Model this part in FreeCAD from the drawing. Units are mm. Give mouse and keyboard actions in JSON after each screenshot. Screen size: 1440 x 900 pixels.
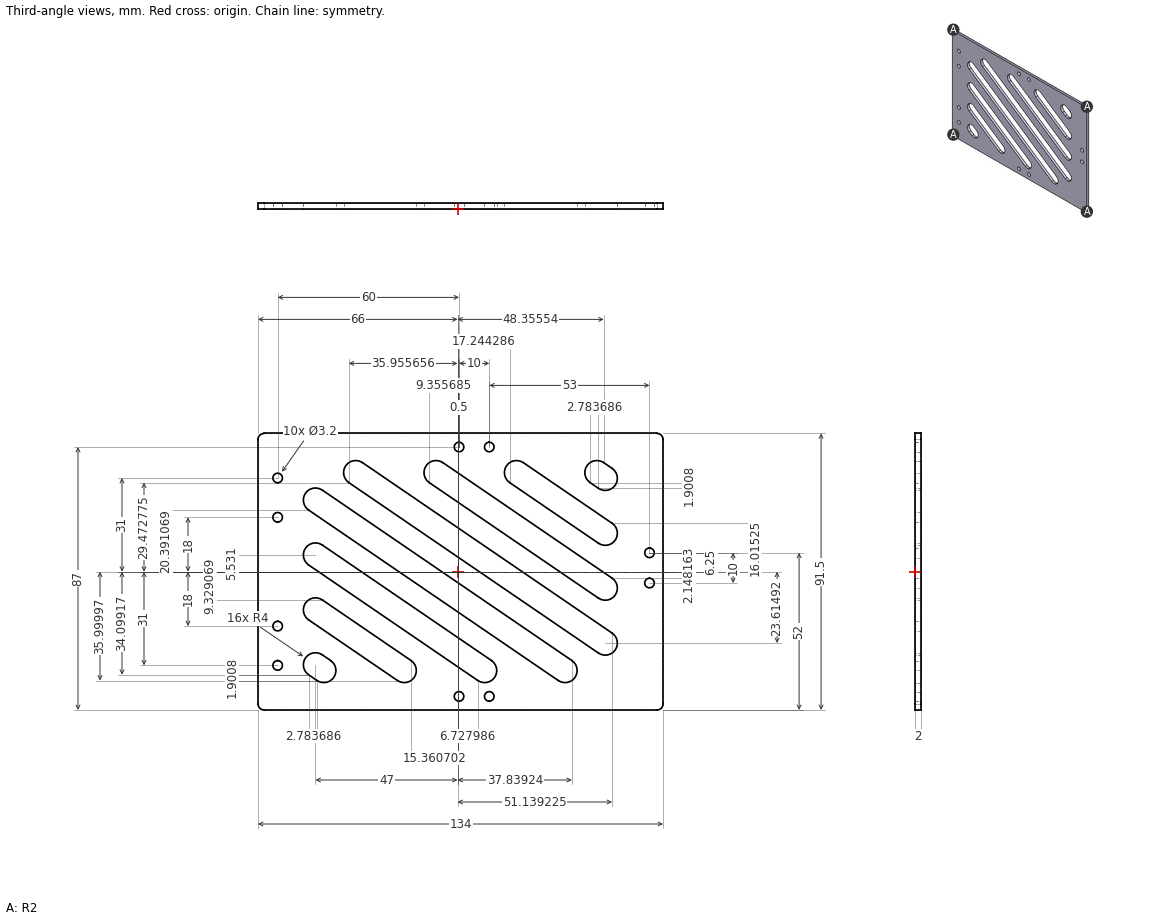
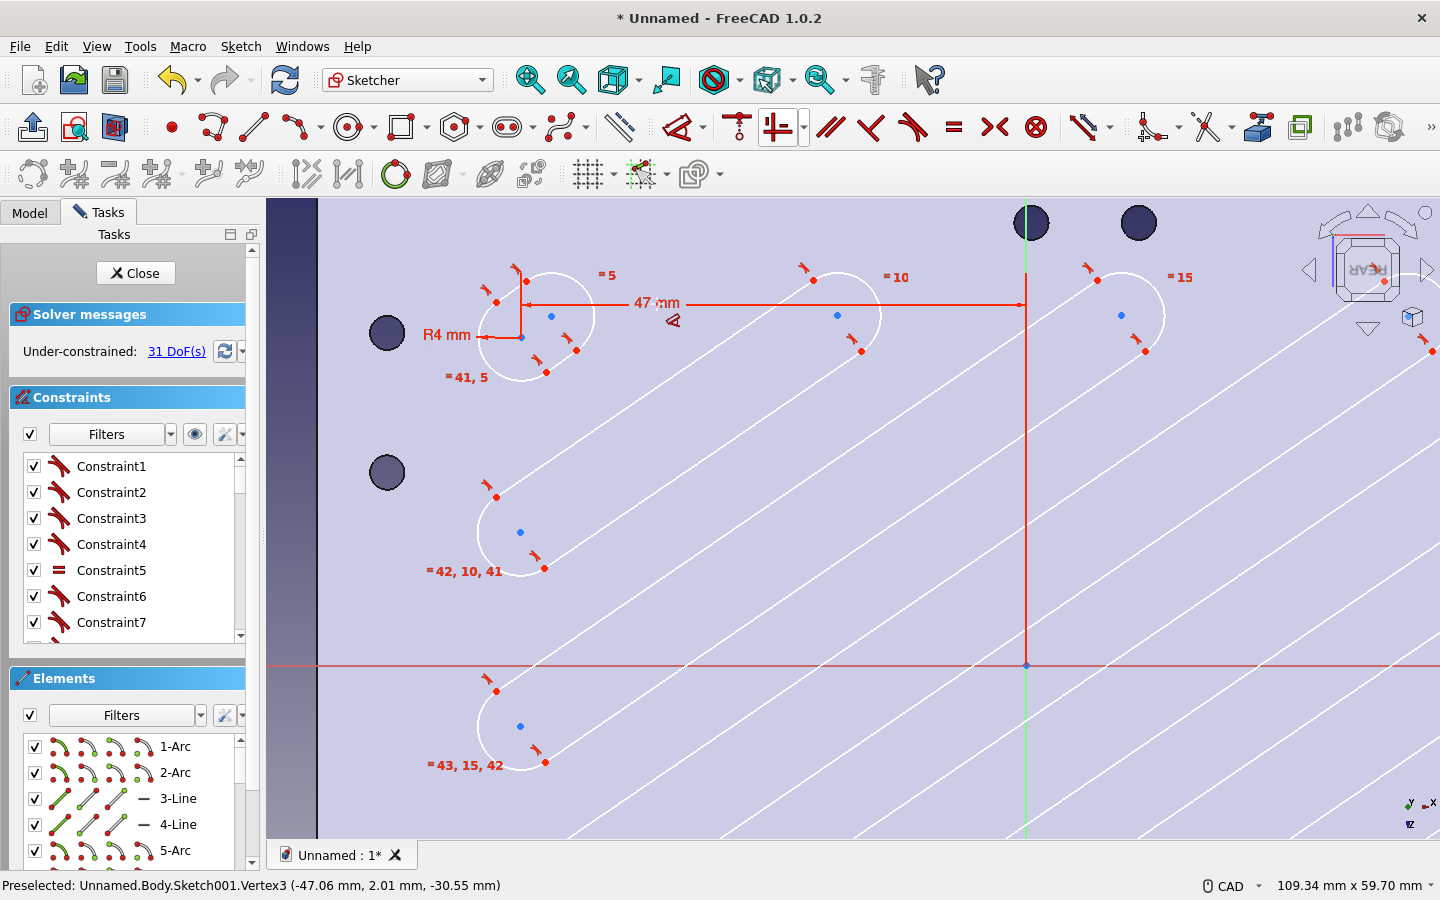
{"action": "left_click", "coordinate": [520, 533]}
{"action": "left_click", "coordinate": [890, 499]}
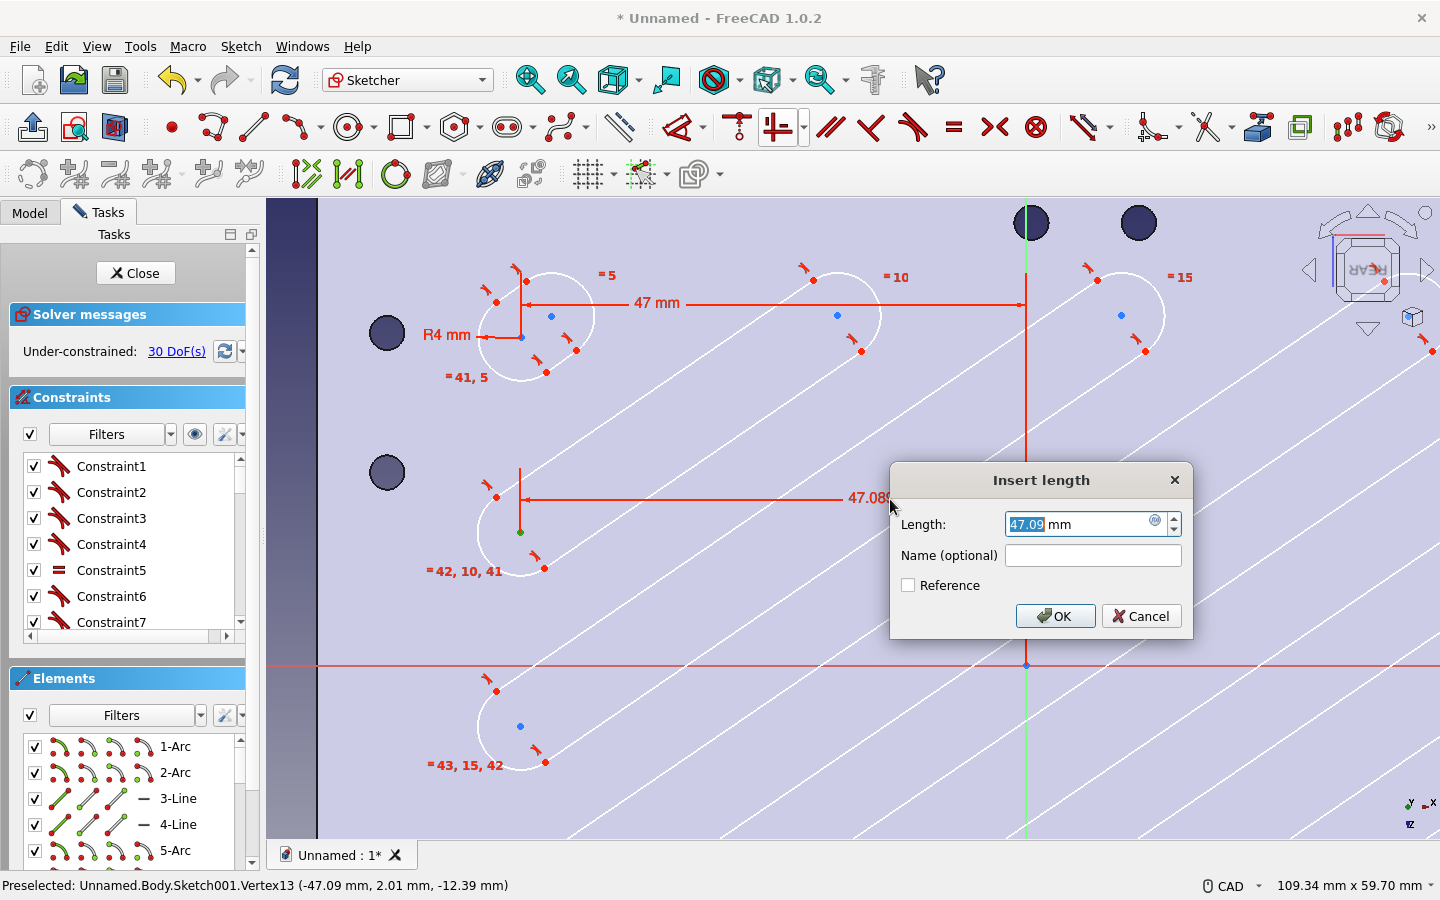
{"action": "type", "text": "47"}
{"action": "key", "text": "Return"}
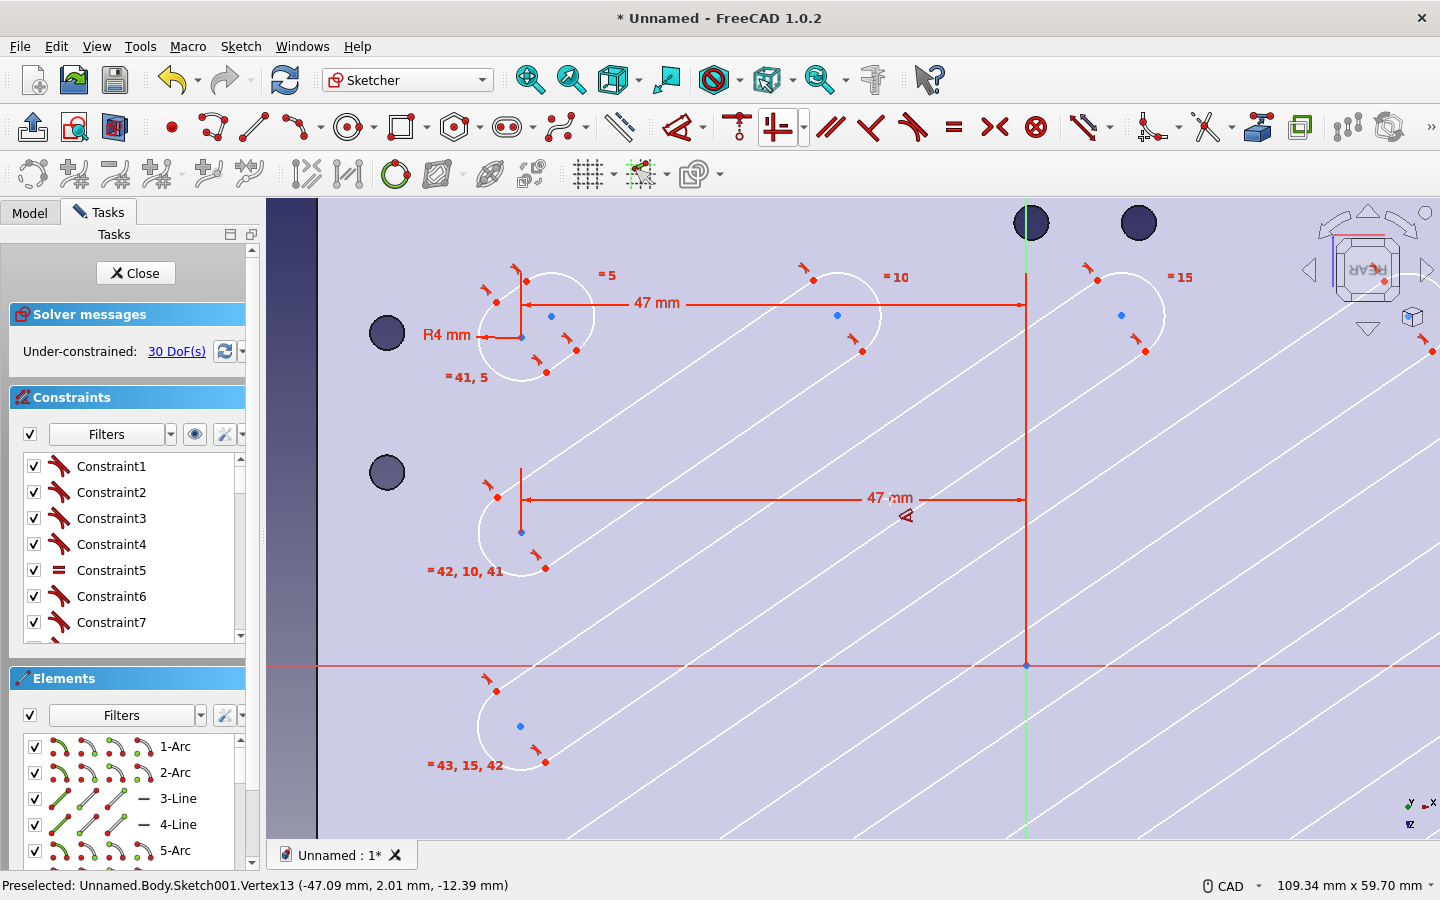
{"action": "left_click", "coordinate": [521, 727]}
{"action": "left_click", "coordinate": [773, 761]}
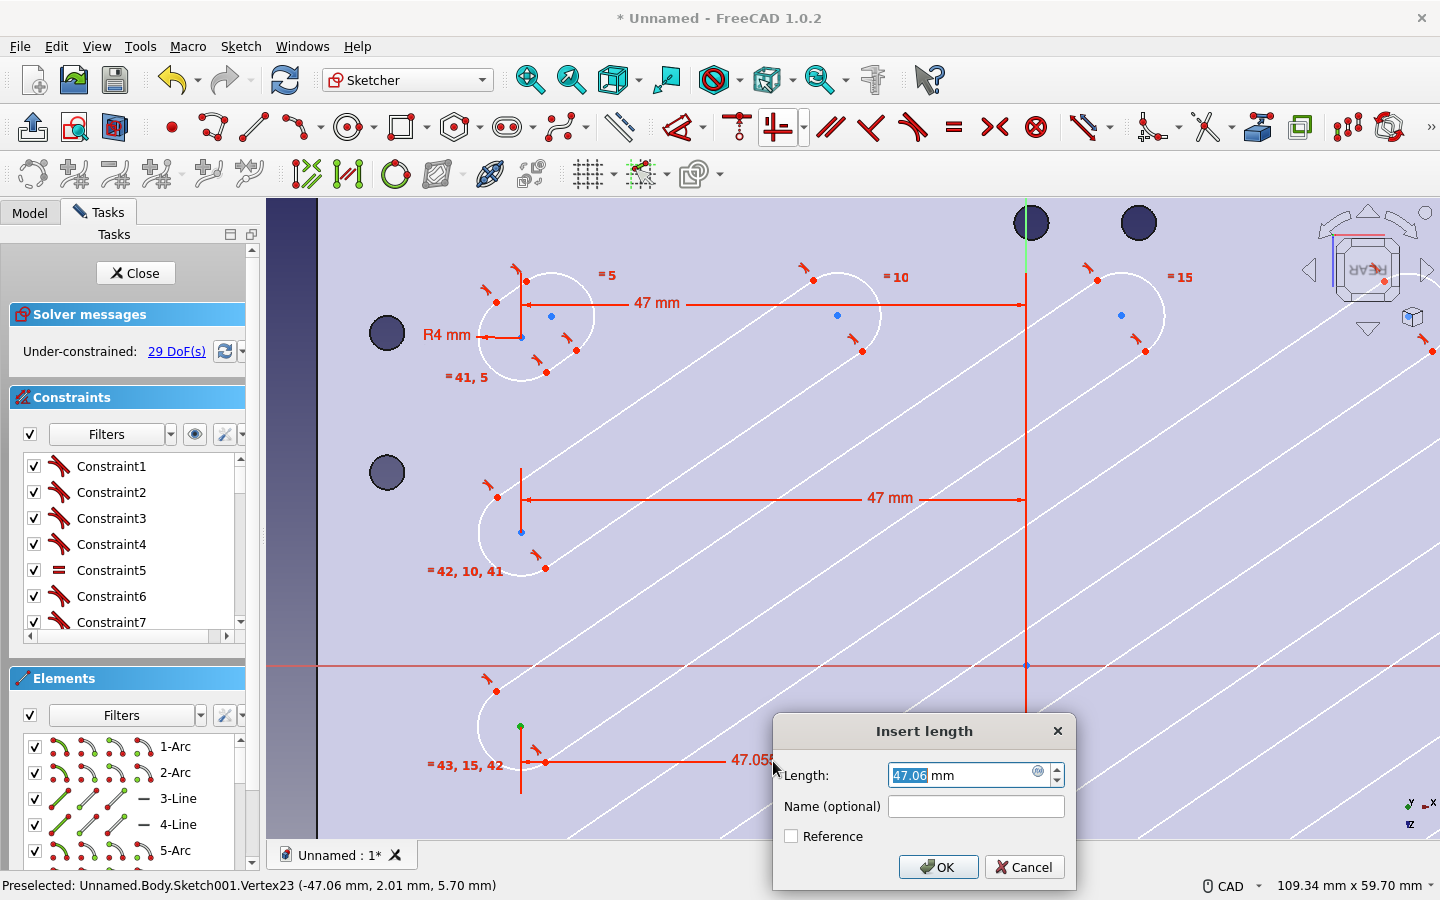
{"action": "type", "text": "47"}
{"action": "key", "text": "Return"}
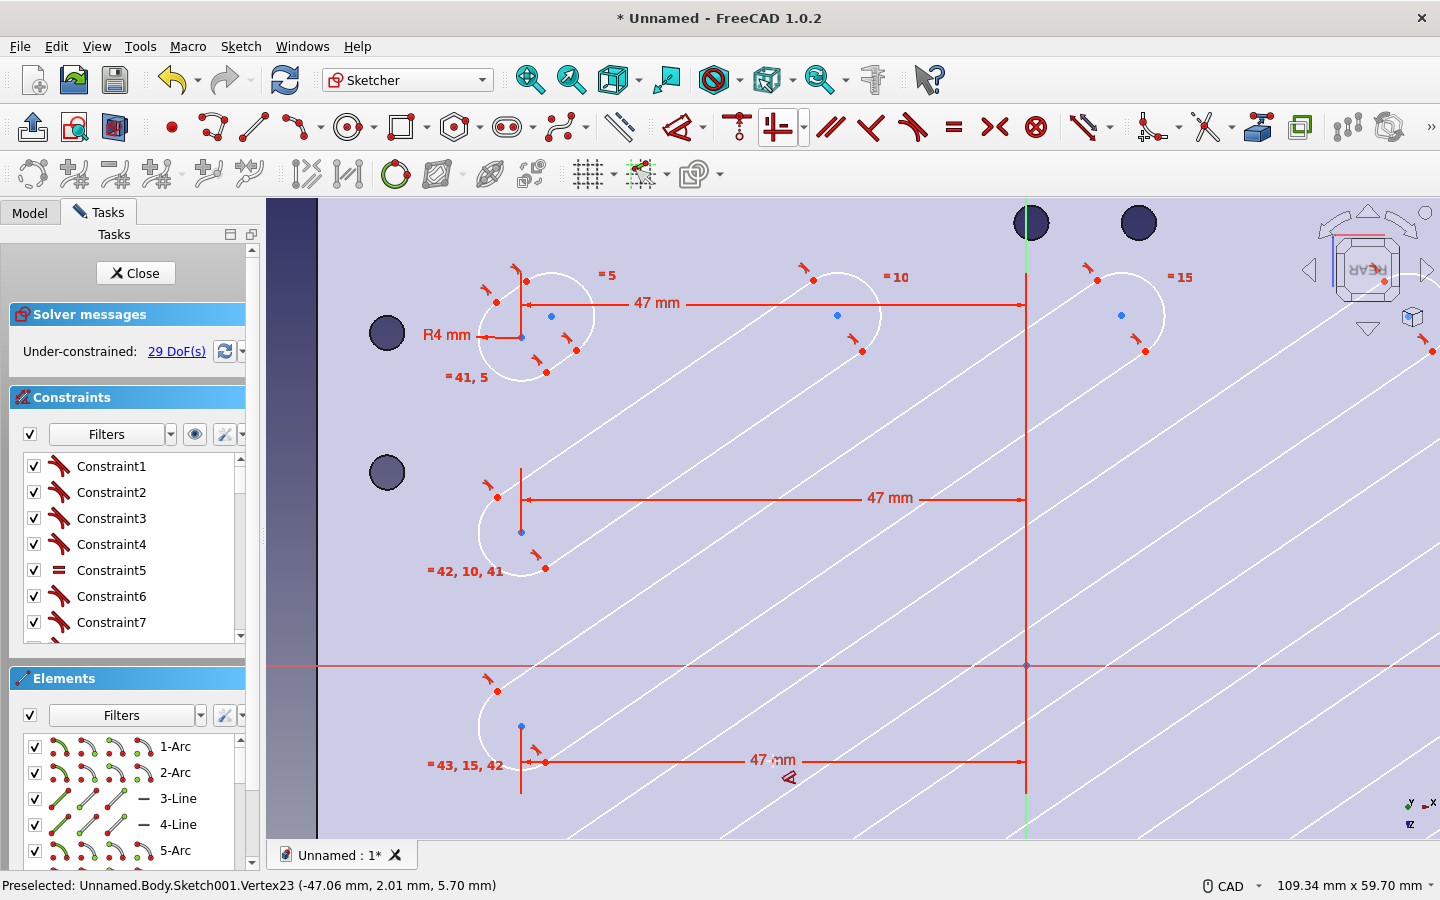
{"action": "scroll", "coordinate": [478, 339], "scroll_direction": "down", "scroll_amount": 3}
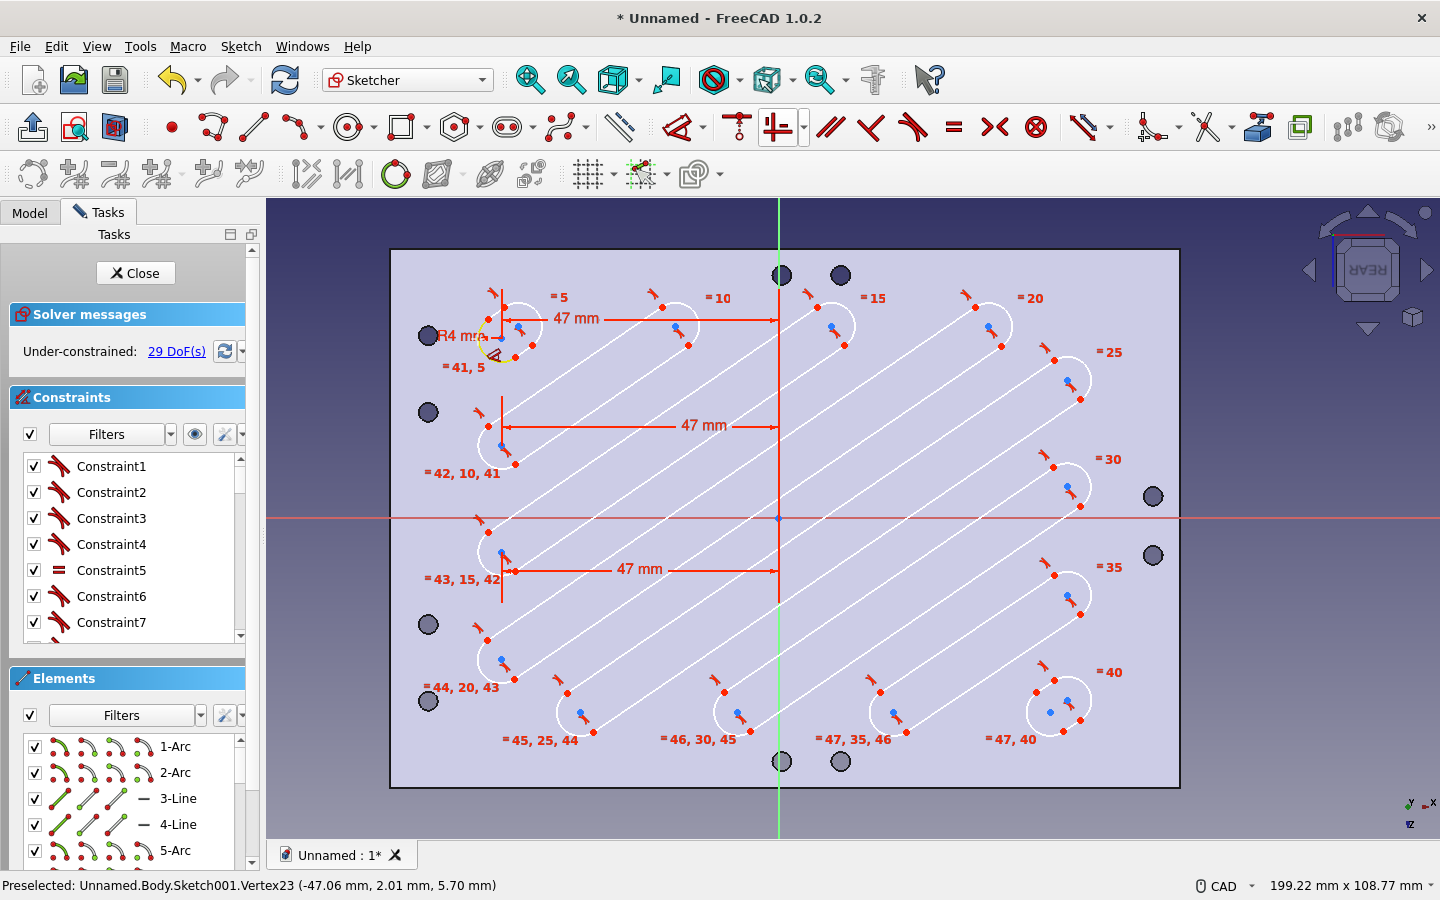
{"action": "left_click", "coordinate": [501, 660]}
{"action": "left_click", "coordinate": [704, 694]}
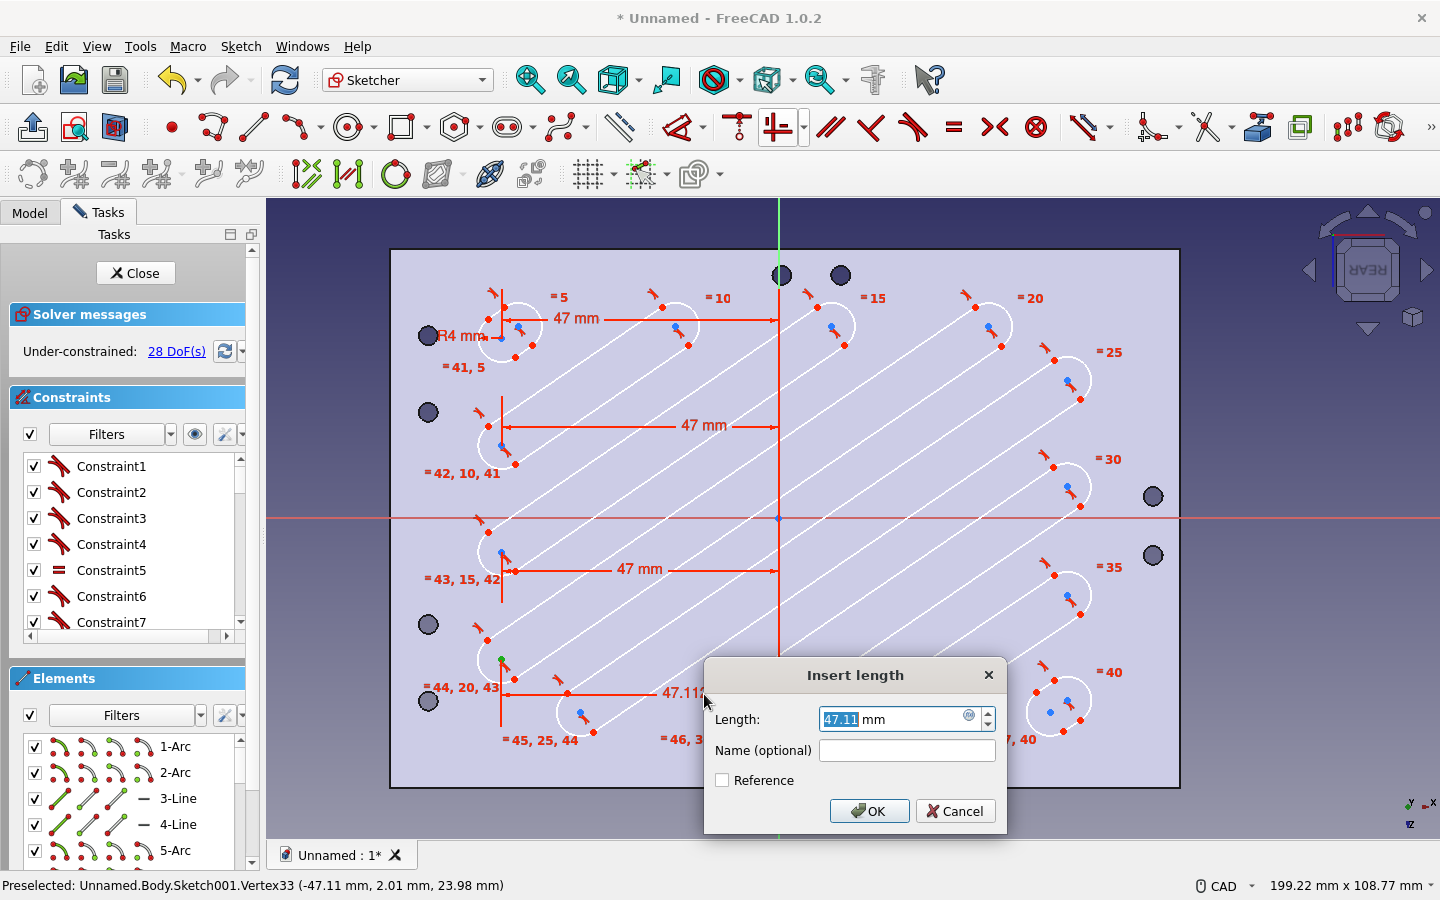
{"action": "type", "text": "47"}
{"action": "key", "text": "Return"}